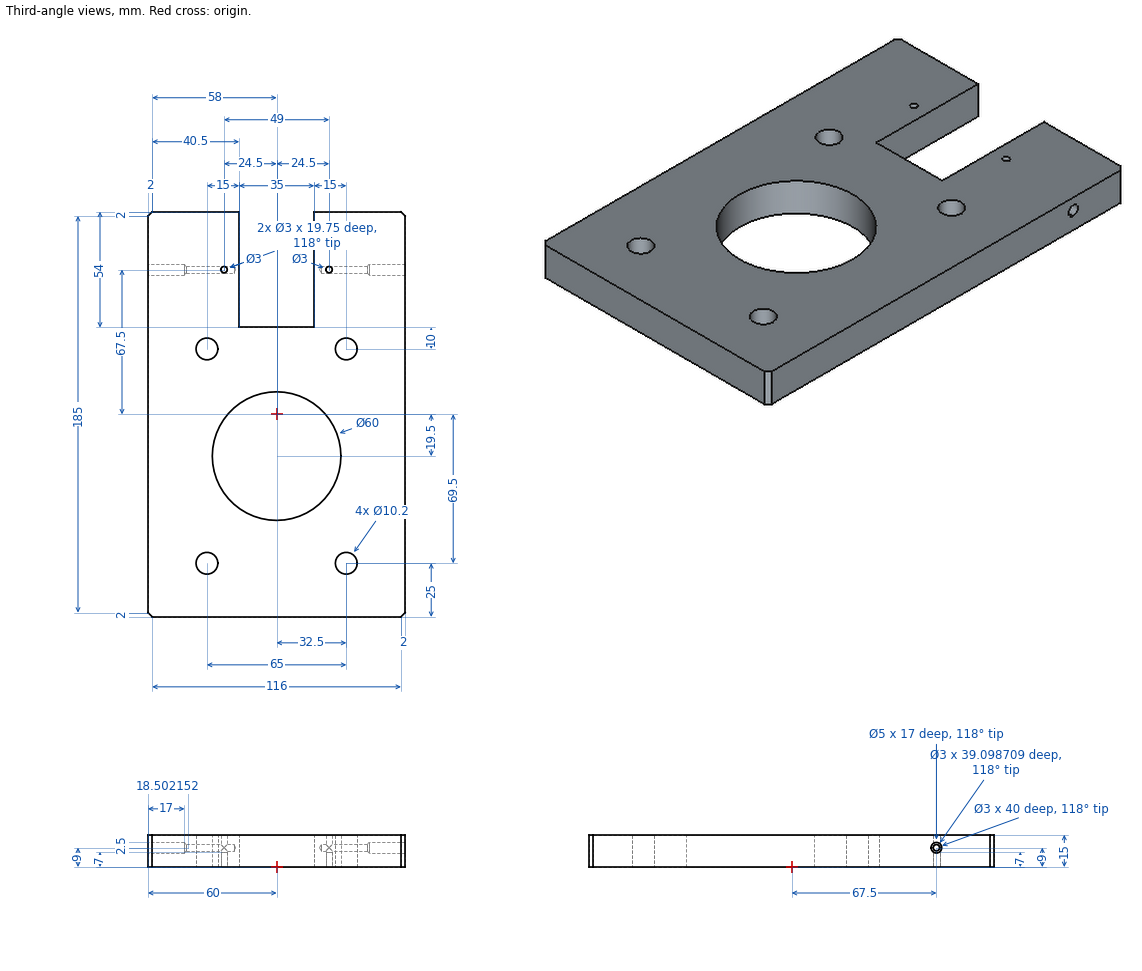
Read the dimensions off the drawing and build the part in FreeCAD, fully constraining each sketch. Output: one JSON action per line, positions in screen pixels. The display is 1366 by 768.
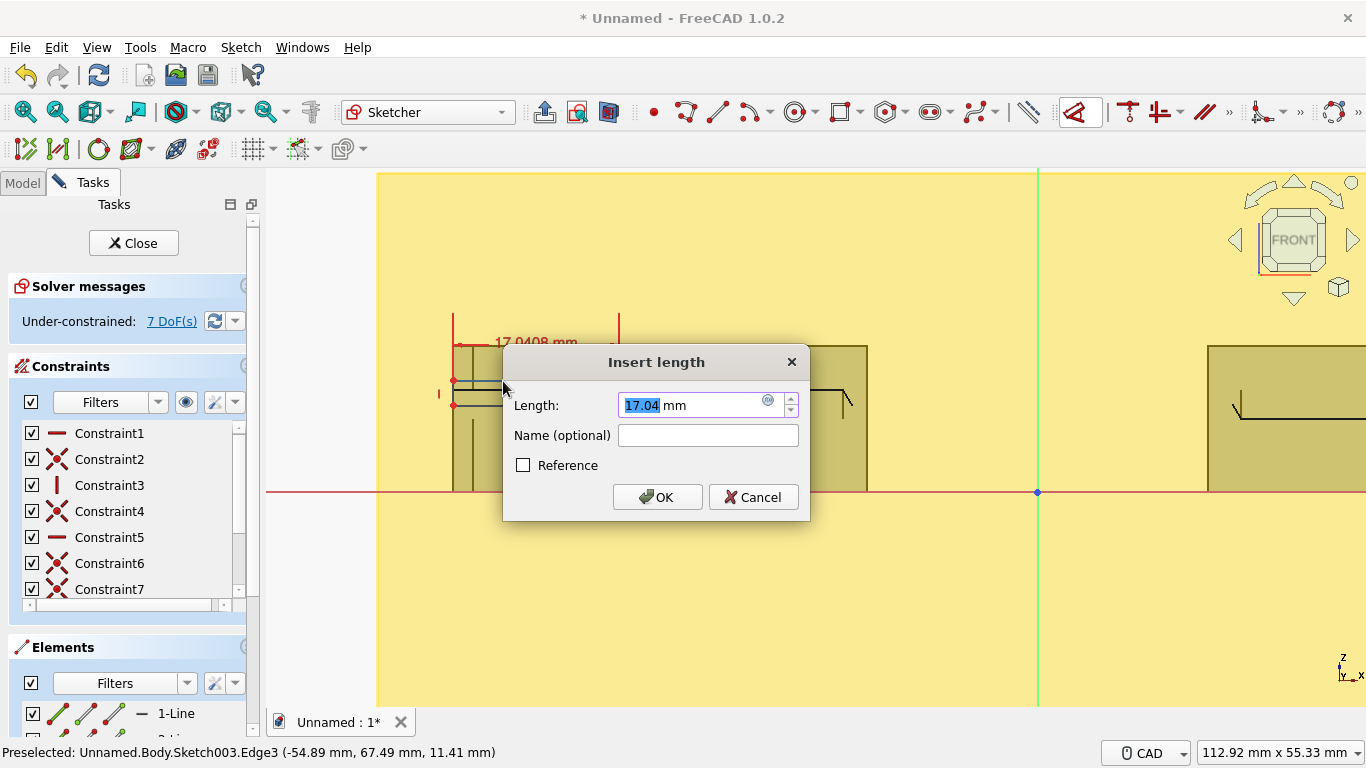
{"action": "type", "text": "17"}
{"action": "key", "text": "Return"}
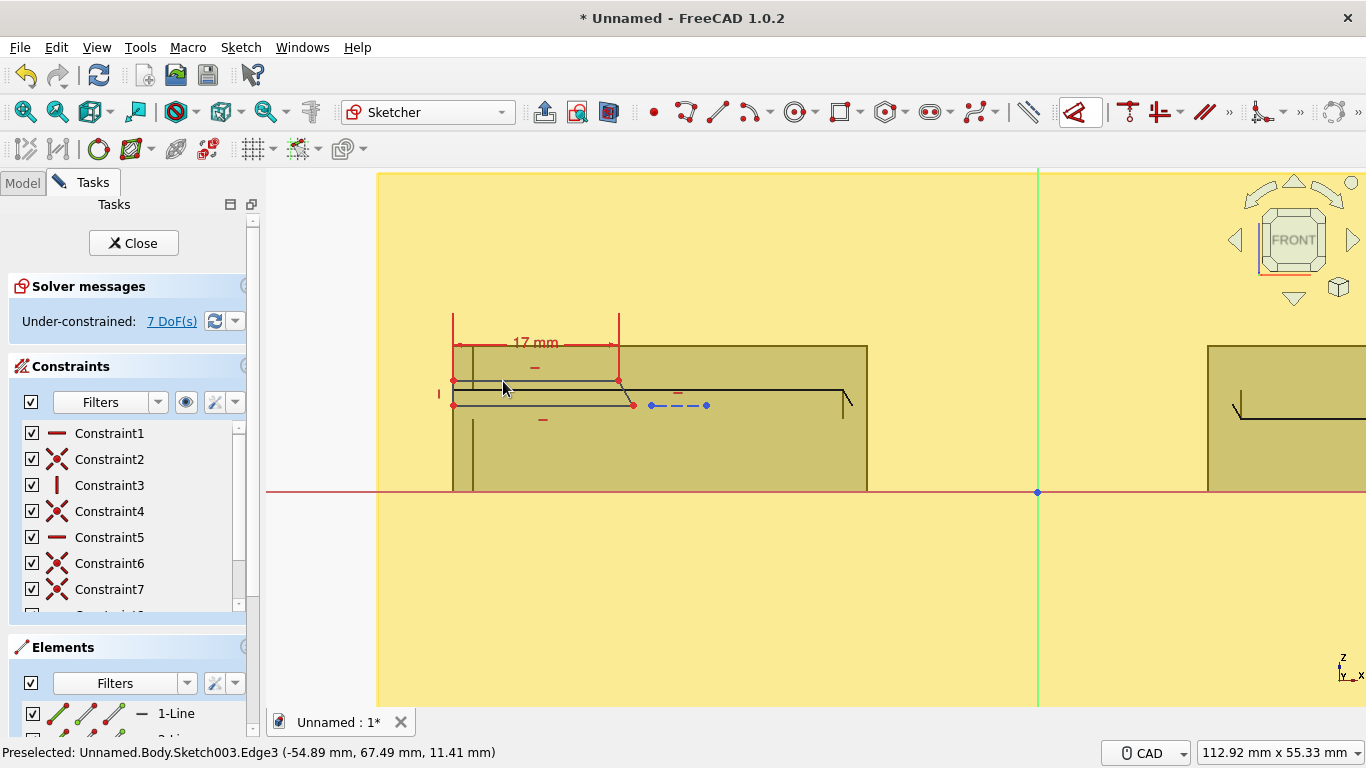
{"action": "left_click", "coordinate": [633, 406]}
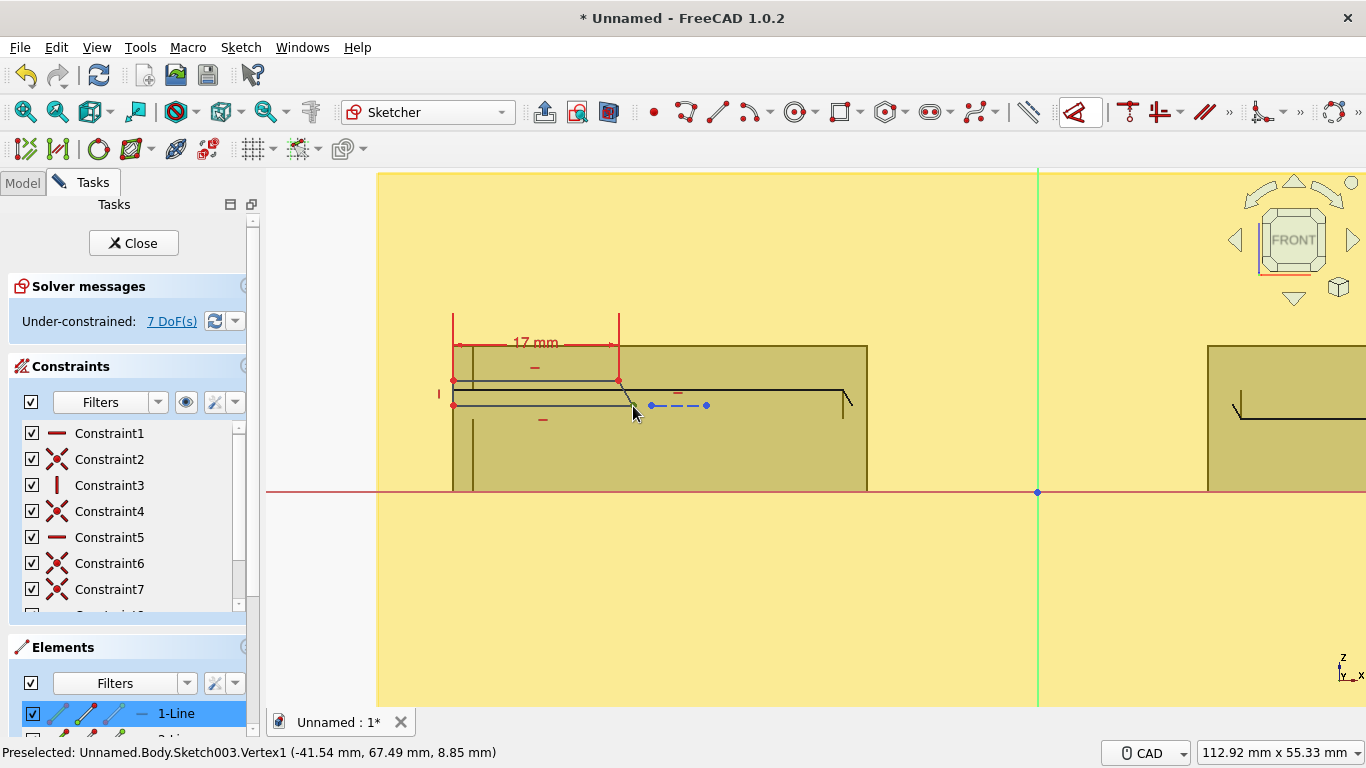
{"action": "key", "text": "i"}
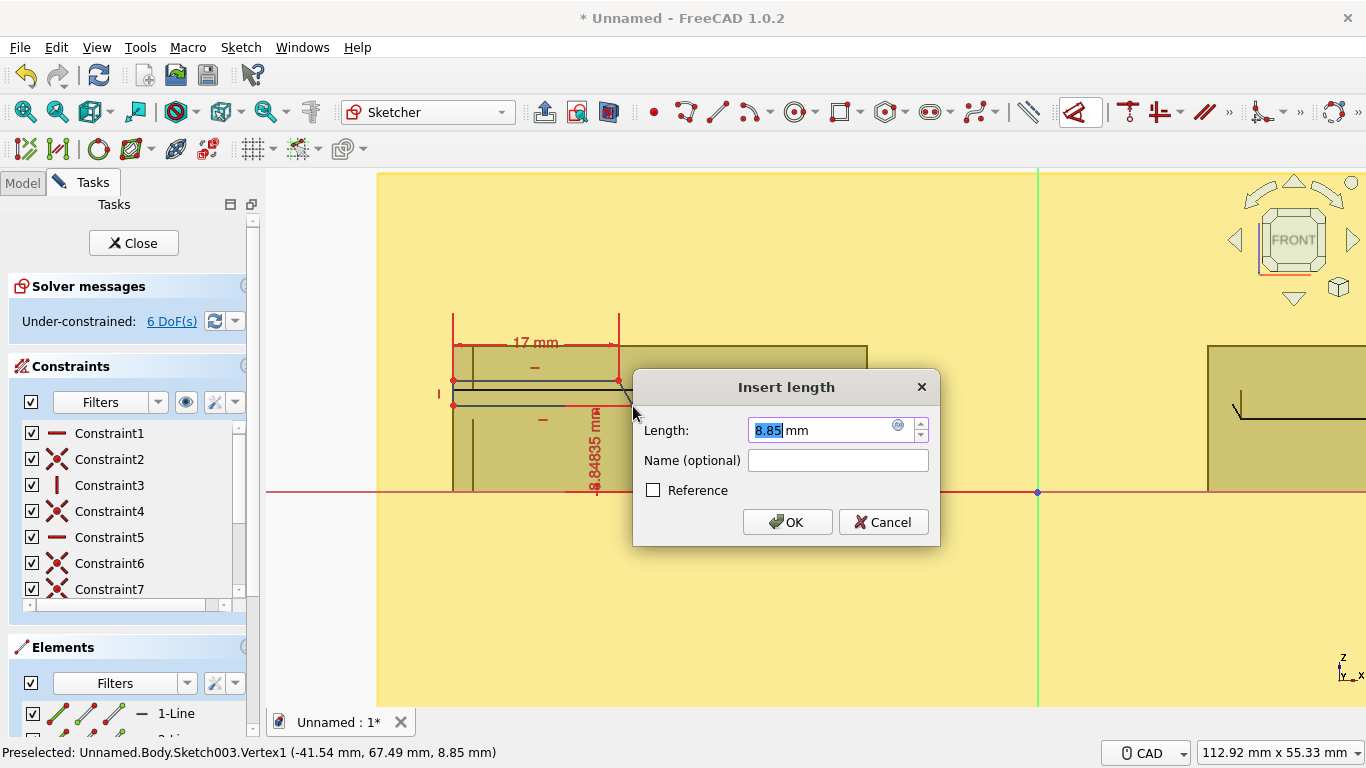
{"action": "type", "text": "9"}
{"action": "key", "text": "Return"}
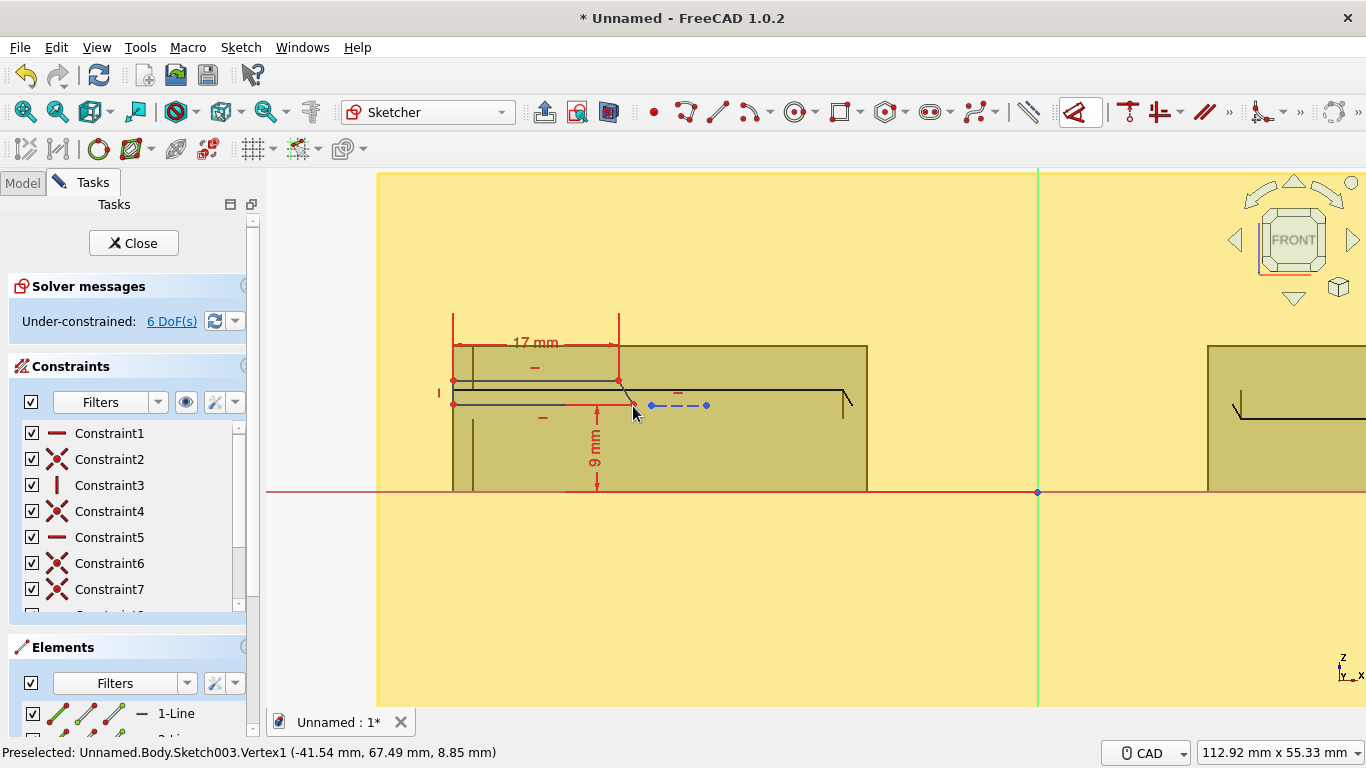
{"action": "left_click", "coordinate": [651, 406]}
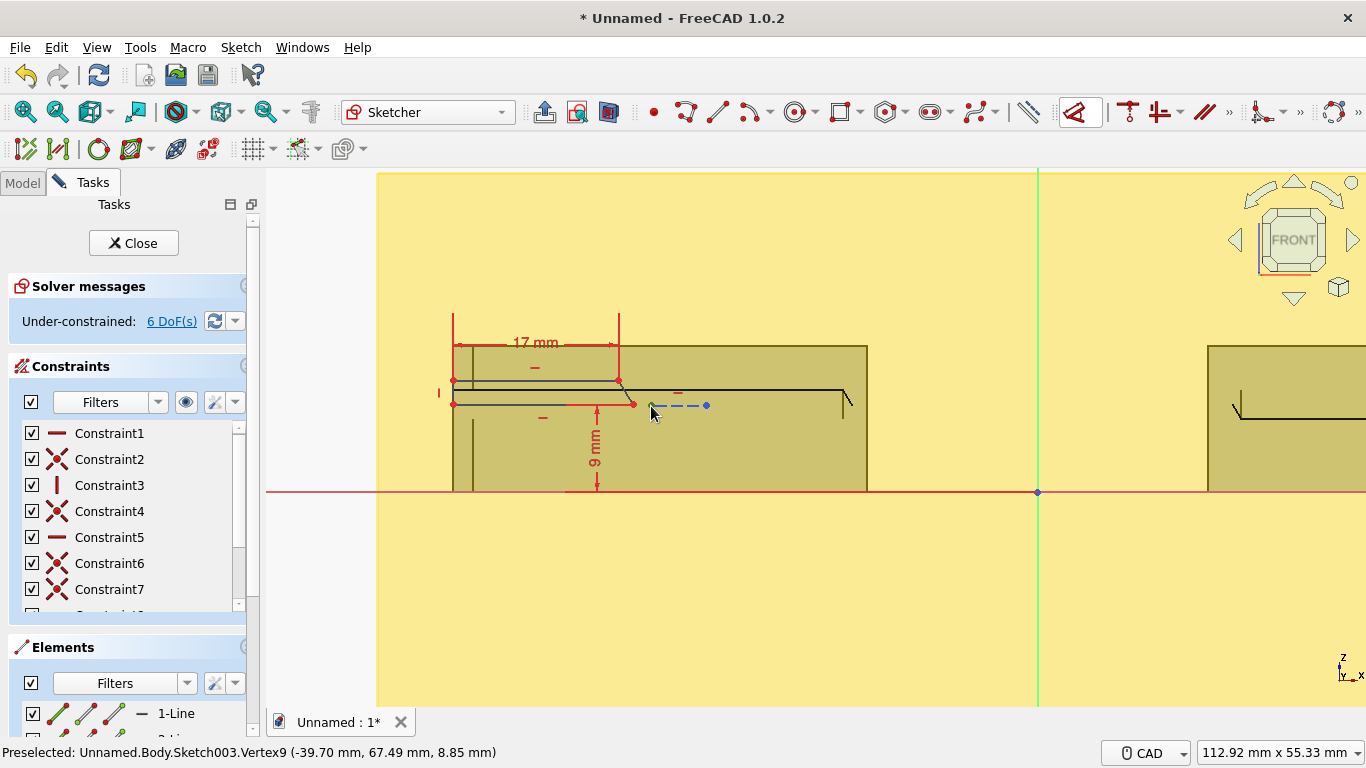
{"action": "left_click", "coordinate": [1096, 112]}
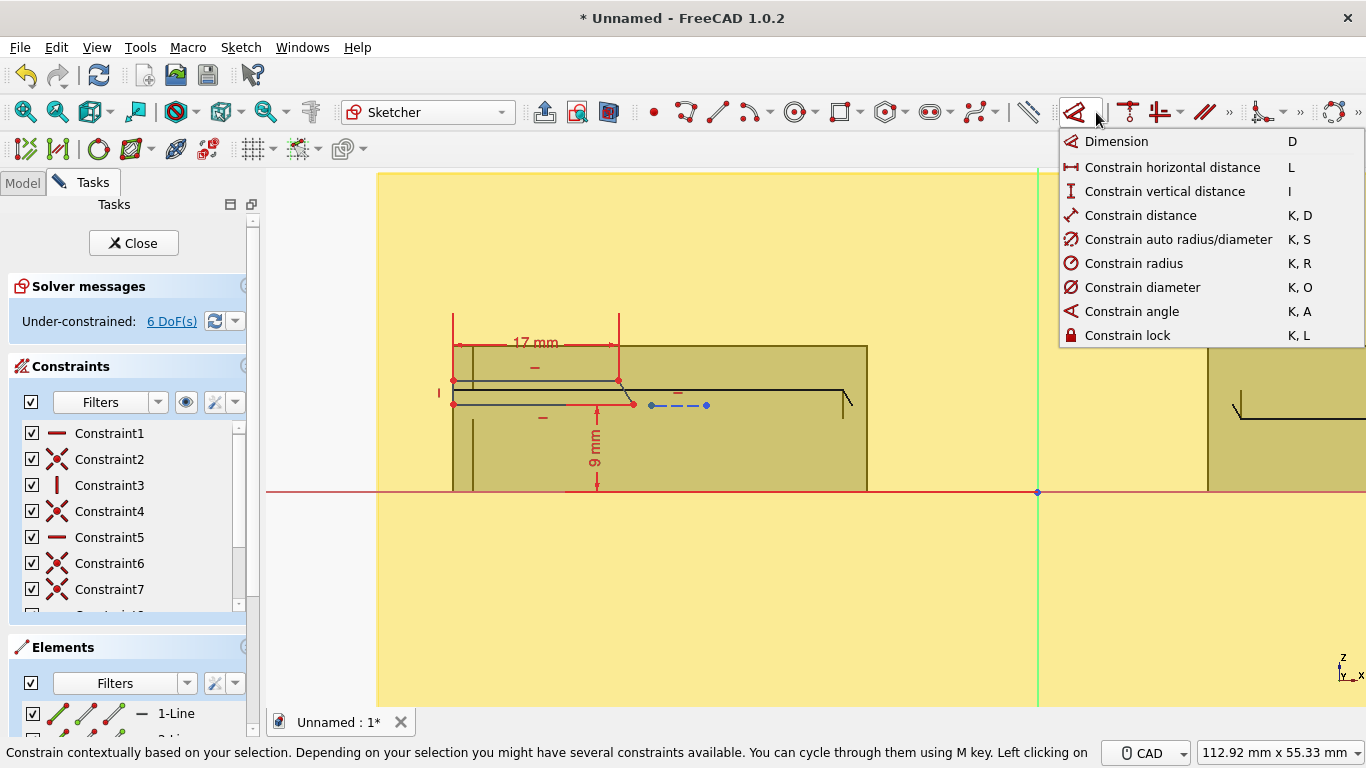
{"action": "left_click", "coordinate": [1212, 191]}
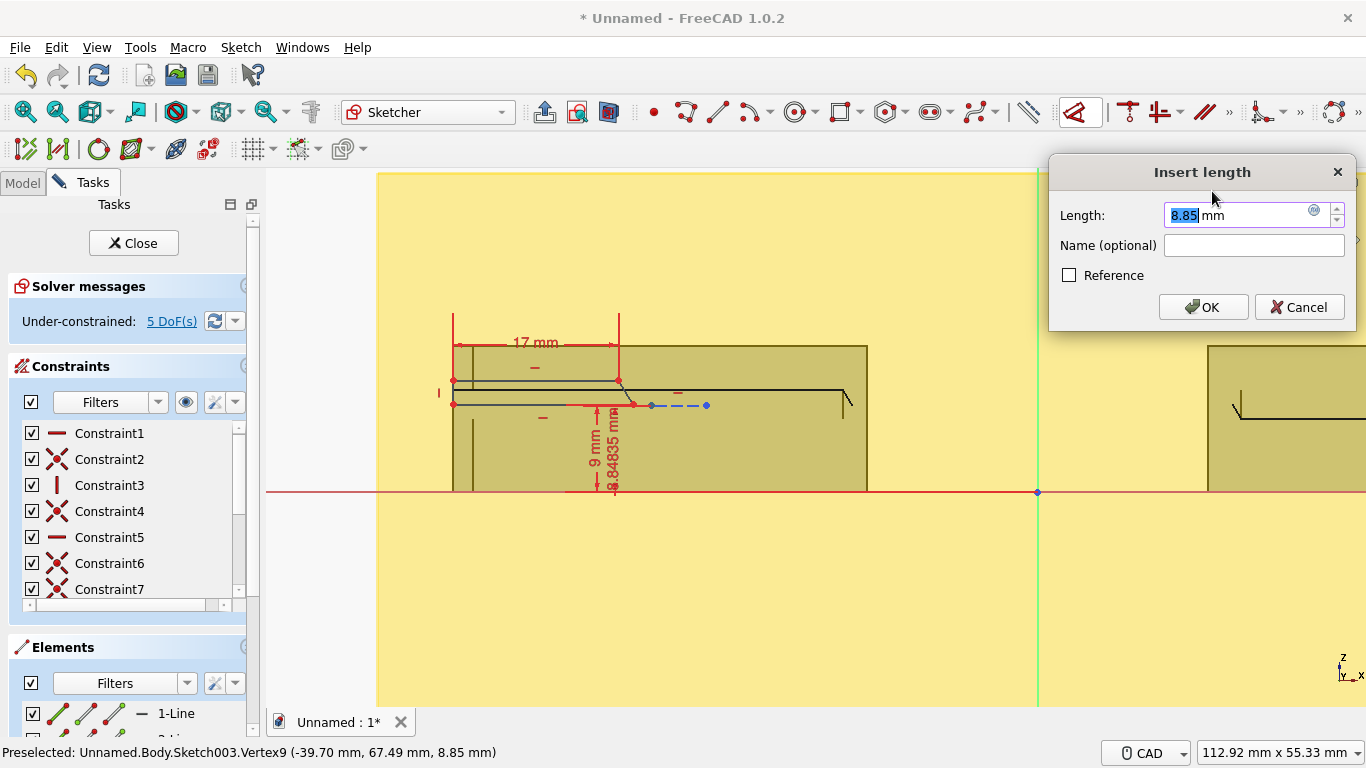
{"action": "type", "text": "9"}
{"action": "key", "text": "Return"}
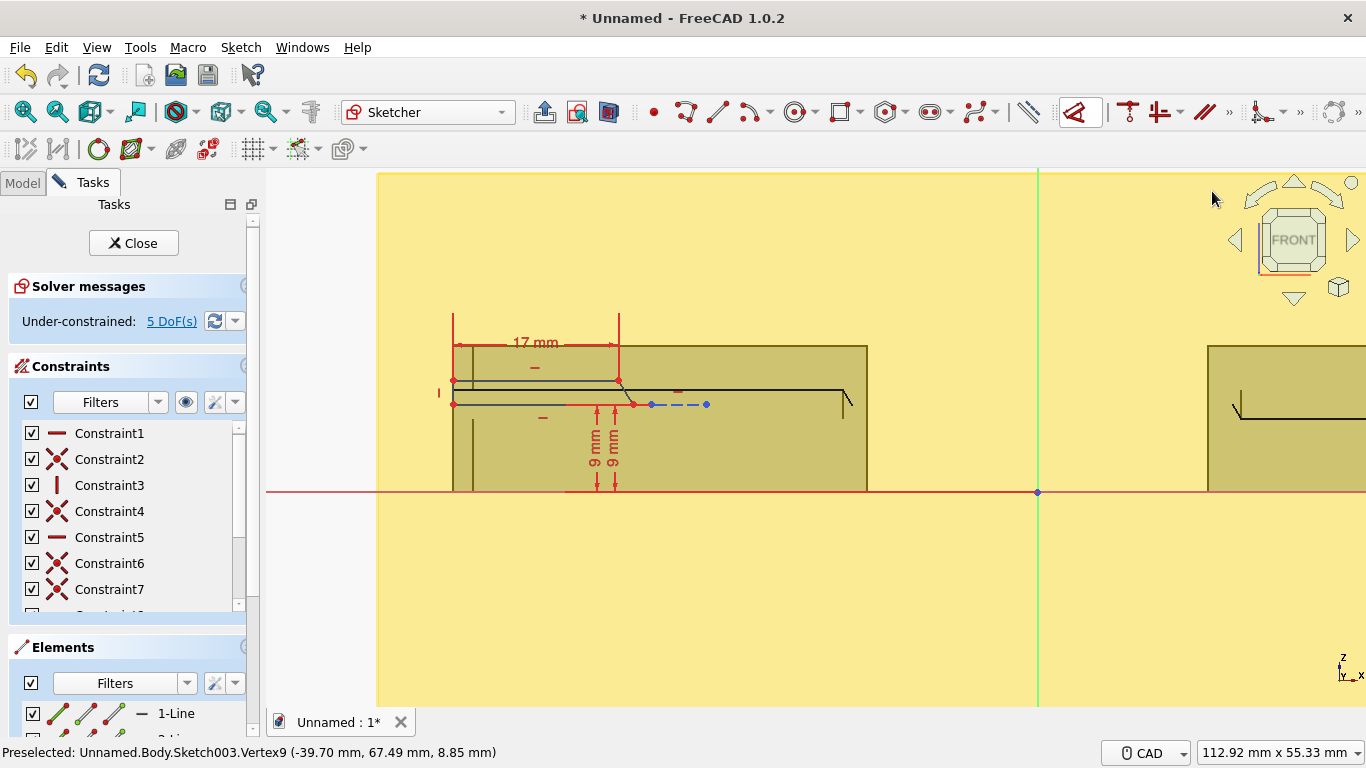
{"action": "scroll", "coordinate": [453, 395], "scroll_direction": "up", "scroll_amount": 3}